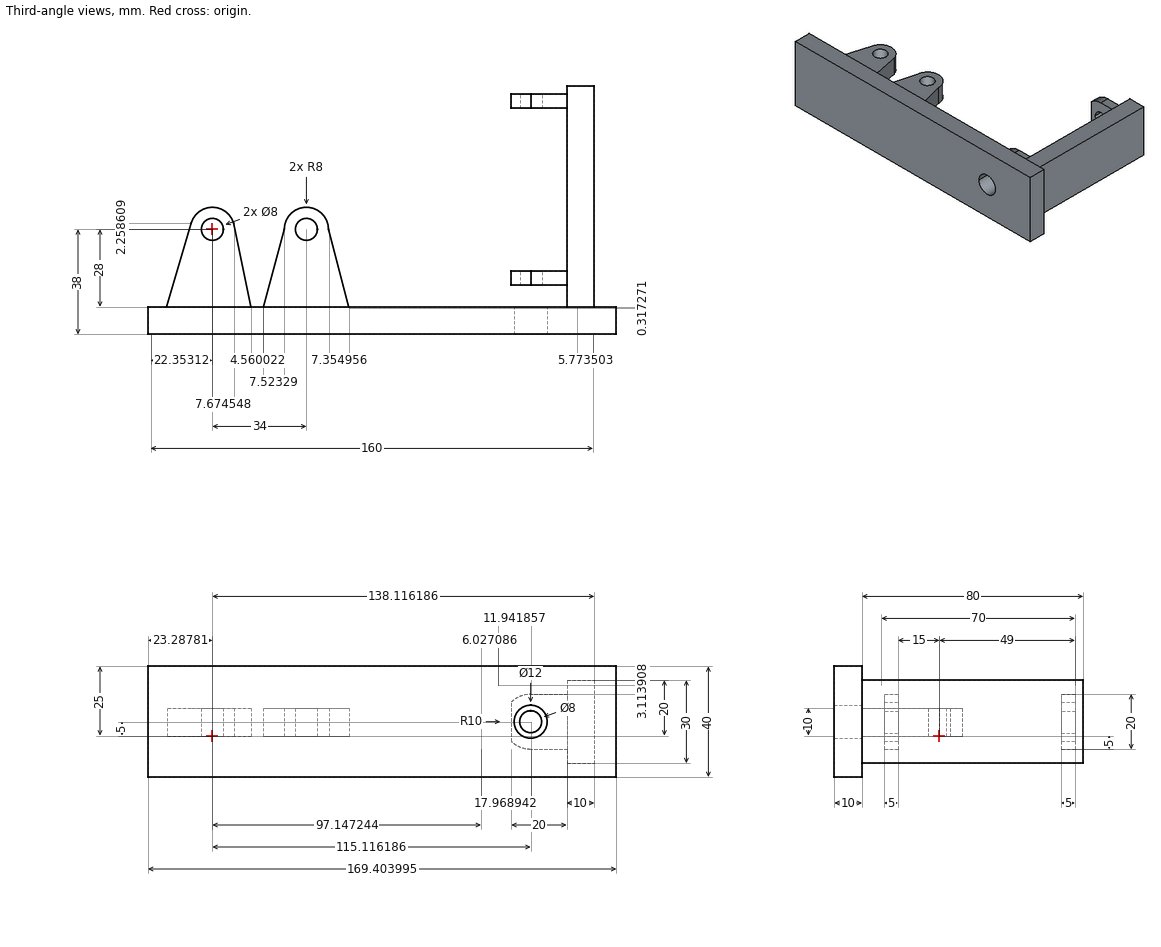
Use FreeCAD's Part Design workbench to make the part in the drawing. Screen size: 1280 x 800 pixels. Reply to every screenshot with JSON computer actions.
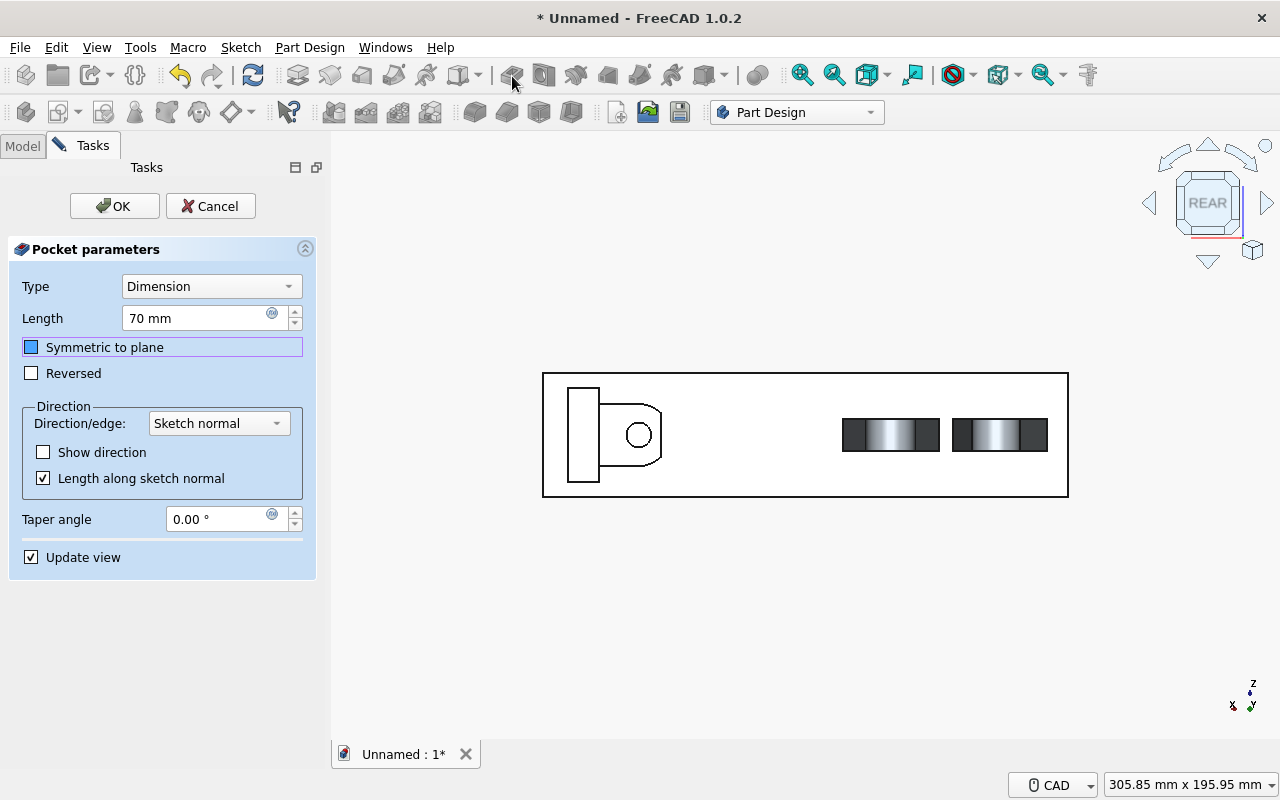
{"action": "left_click", "coordinate": [115, 206]}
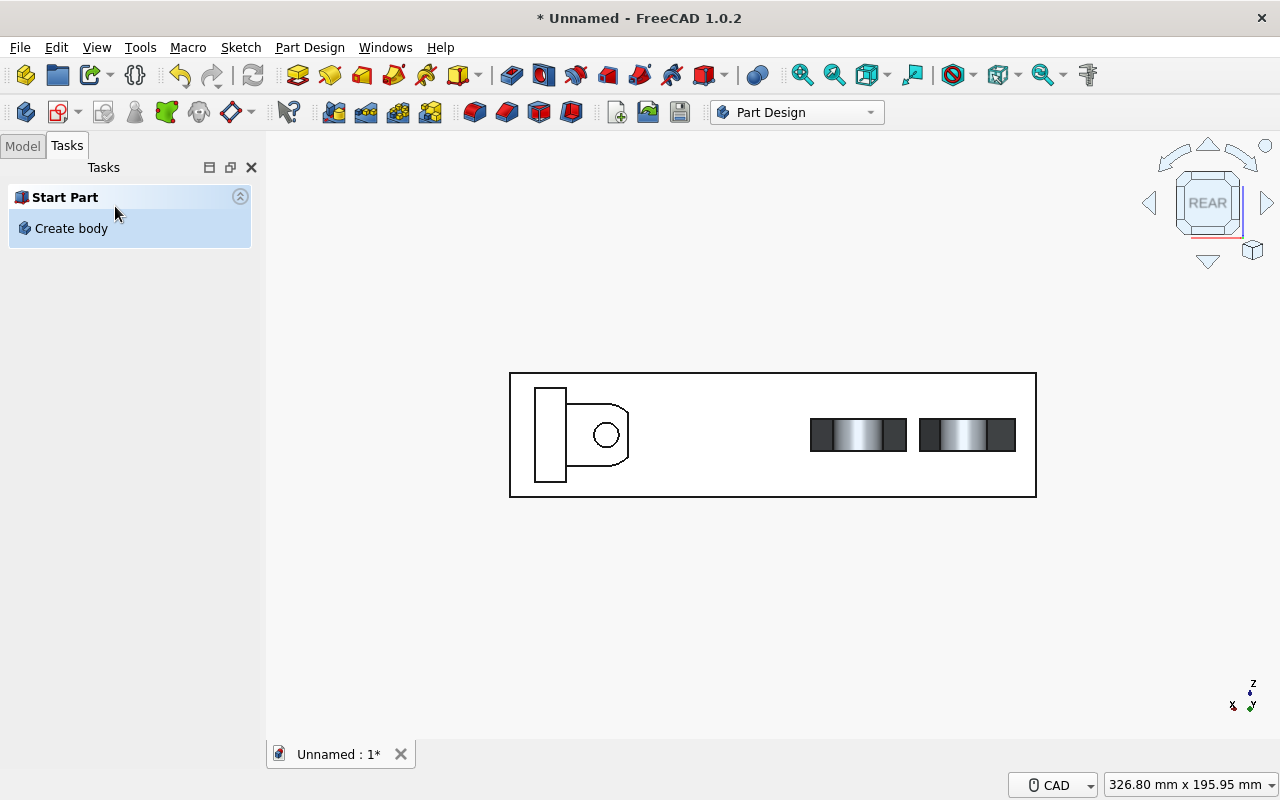
{"action": "left_click", "coordinate": [698, 434]}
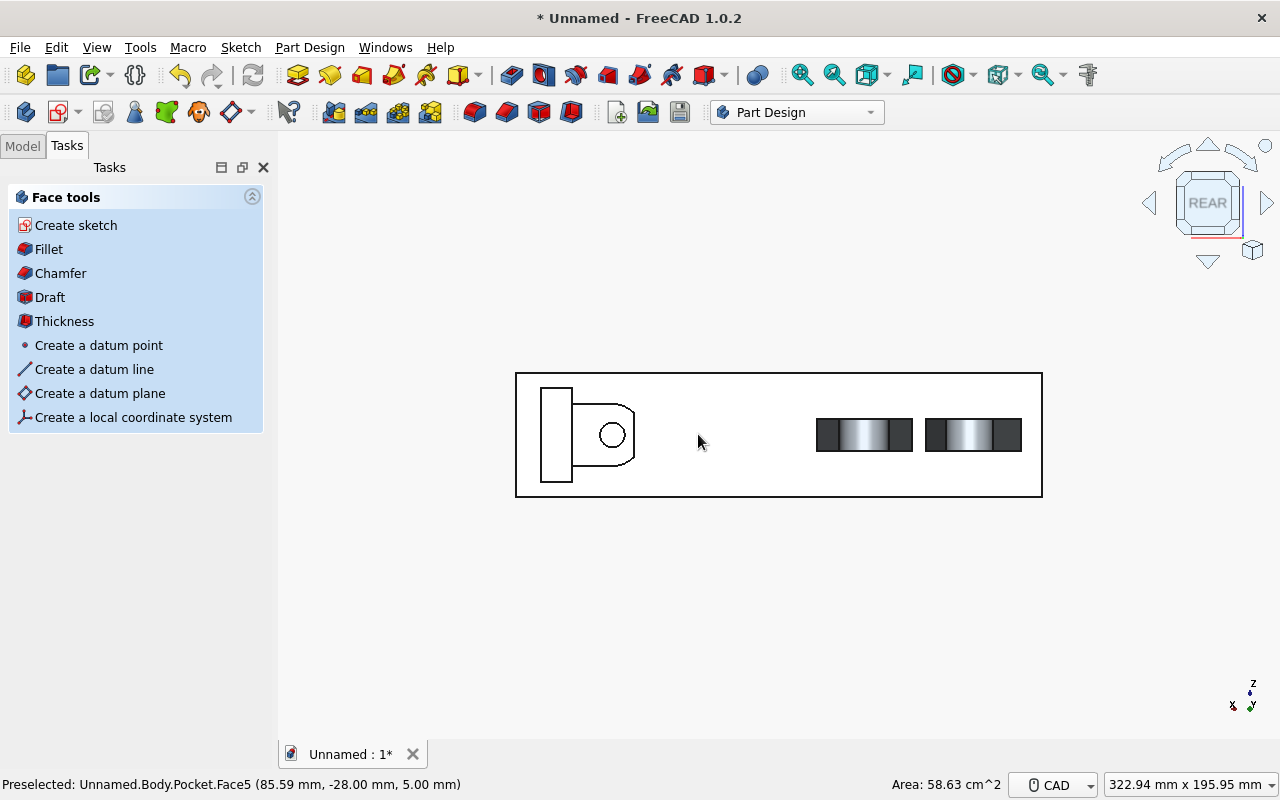
{"action": "left_click", "coordinate": [58, 112]}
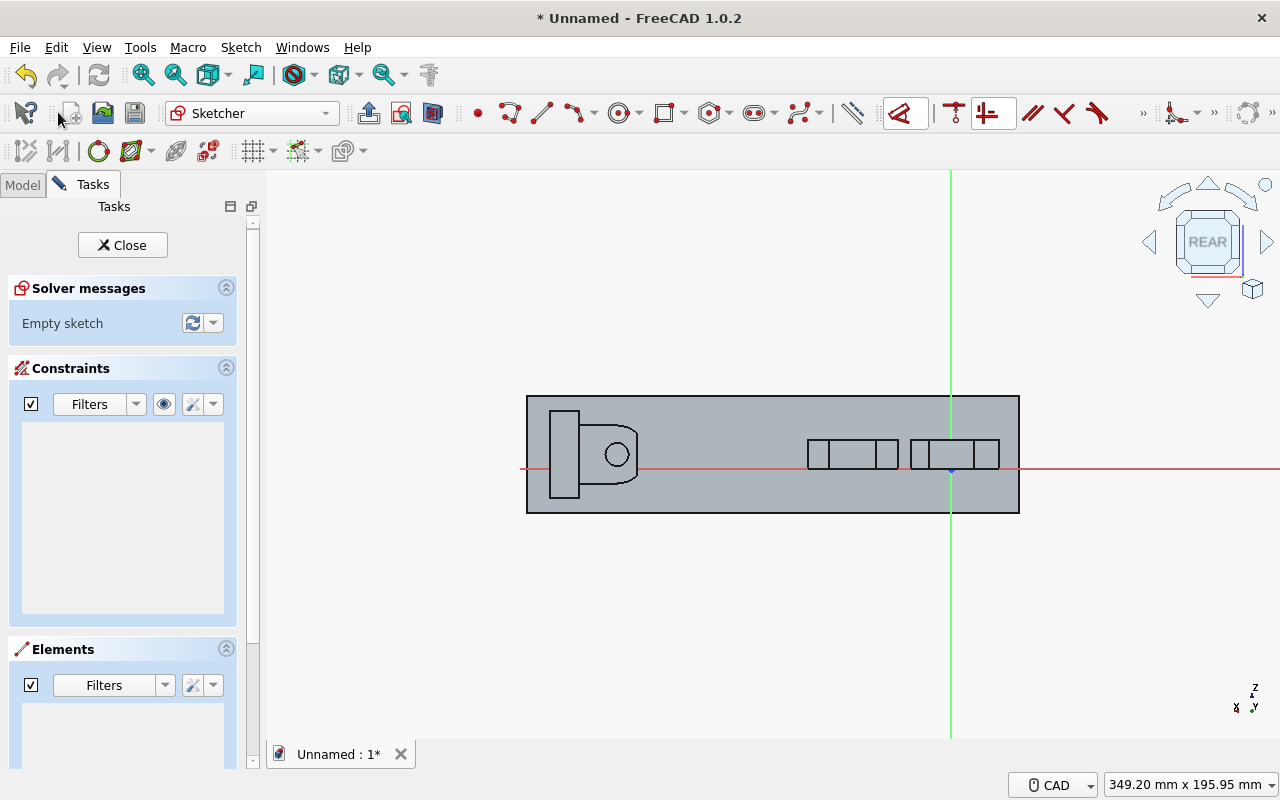
{"action": "scroll", "coordinate": [608, 455], "scroll_direction": "up", "scroll_amount": 12}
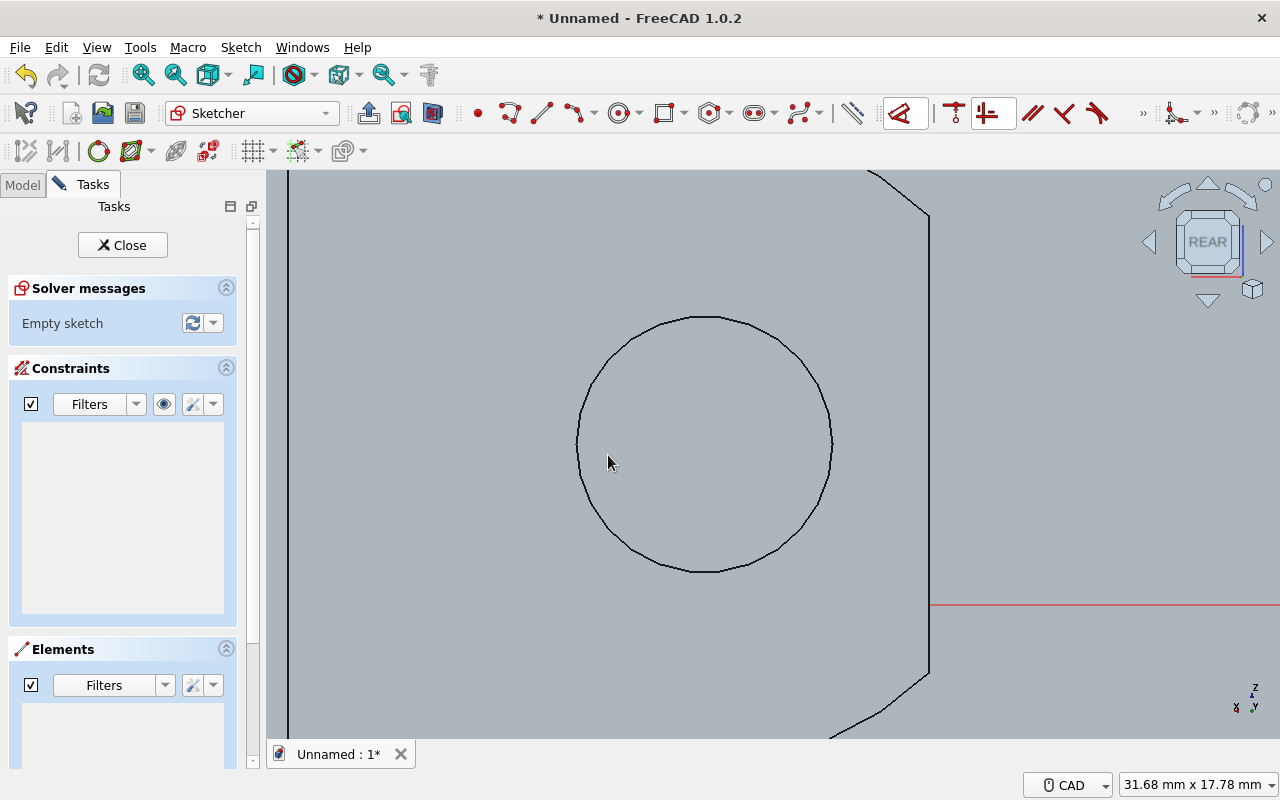
{"action": "left_click", "coordinate": [620, 114]}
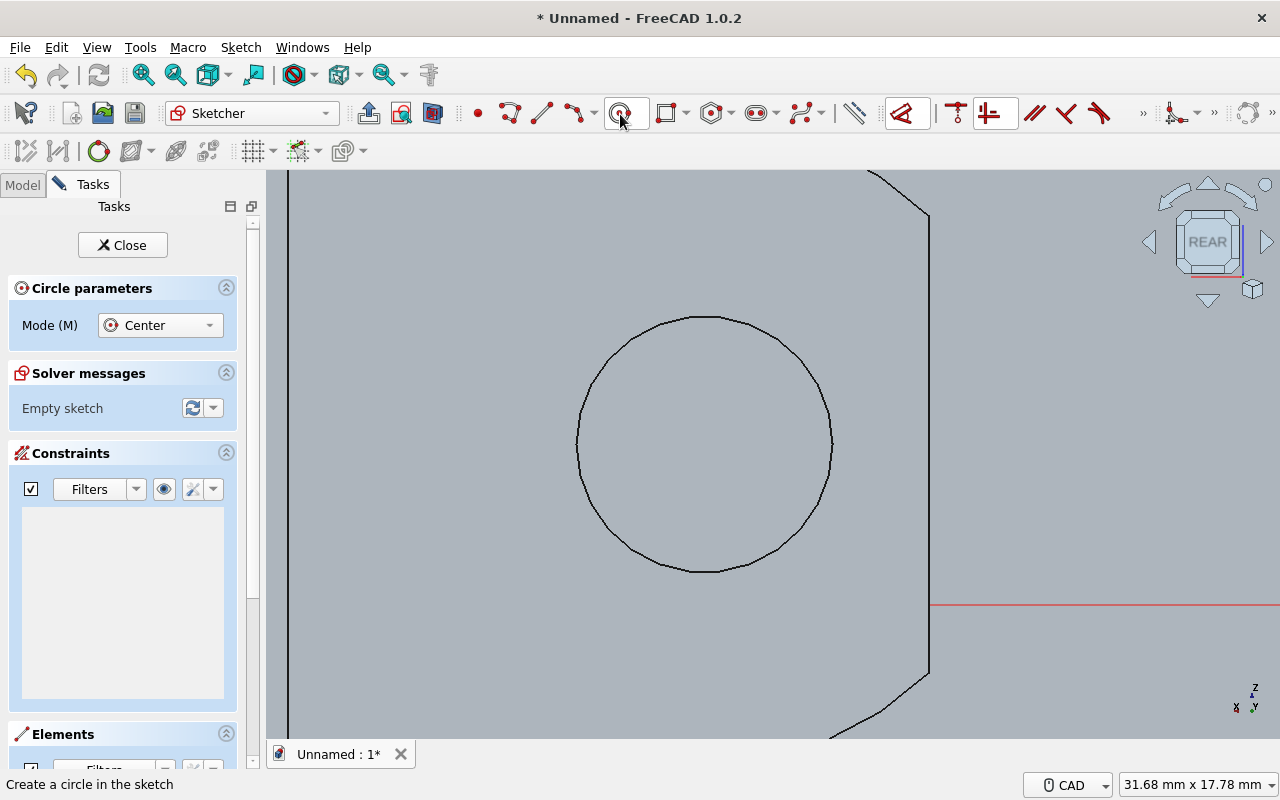
{"action": "left_click", "coordinate": [705, 444]}
{"action": "mouse_move", "coordinate": [840, 309]}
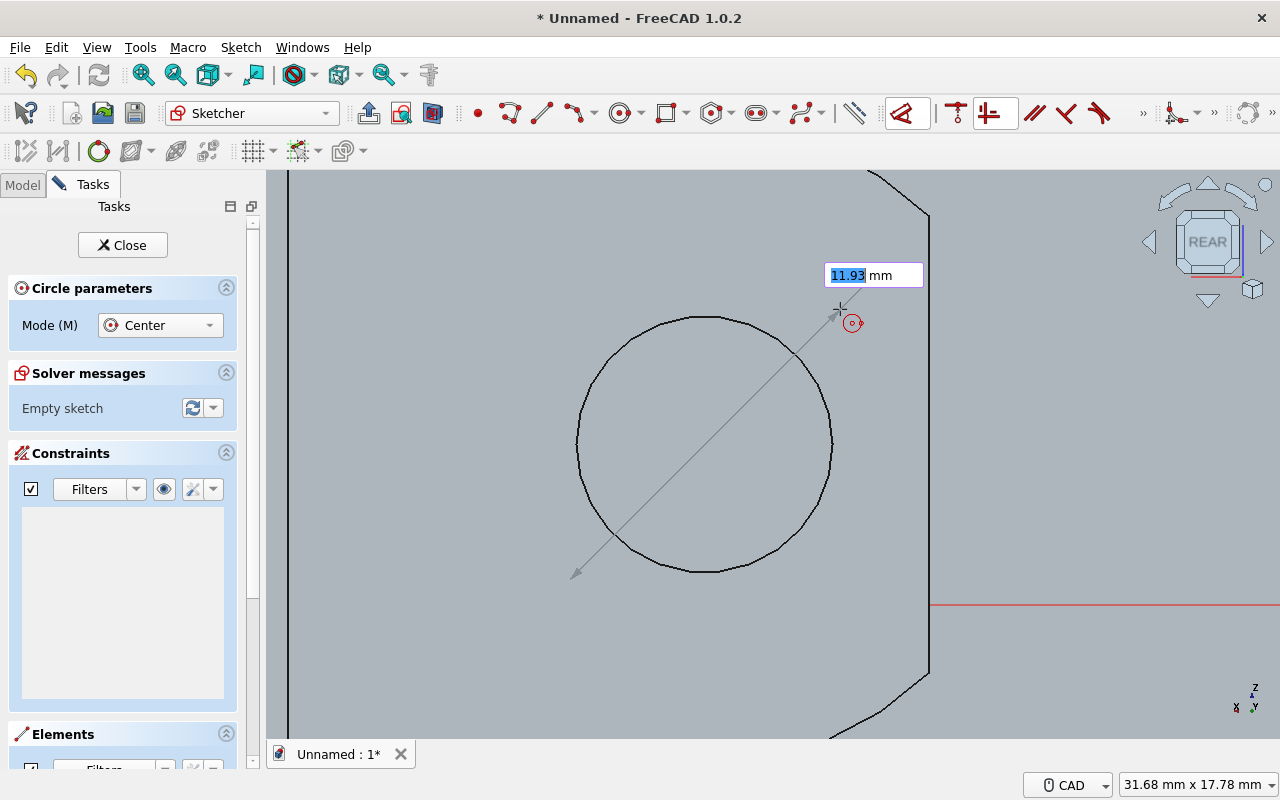
{"action": "type", "text": "12"}
{"action": "key", "text": "Return"}
{"action": "key", "text": "Escape"}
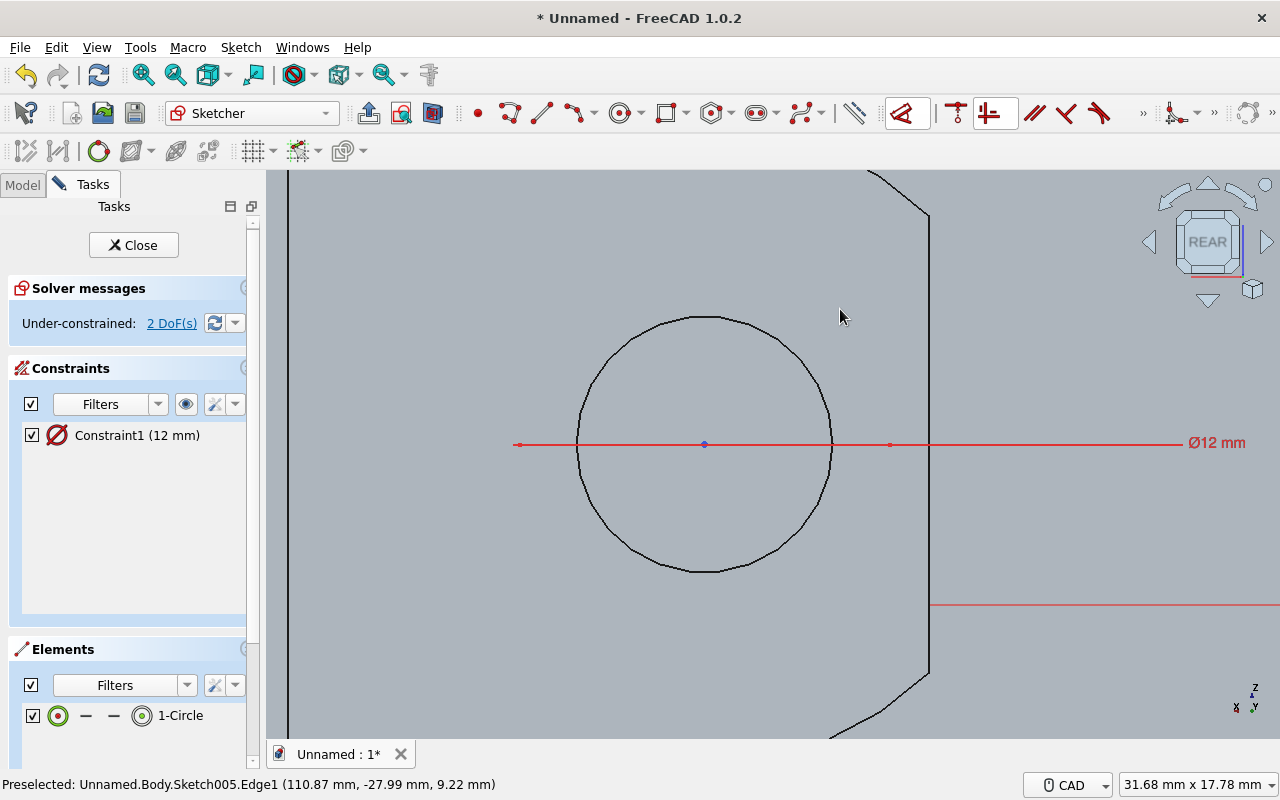
{"action": "left_click", "coordinate": [705, 445]}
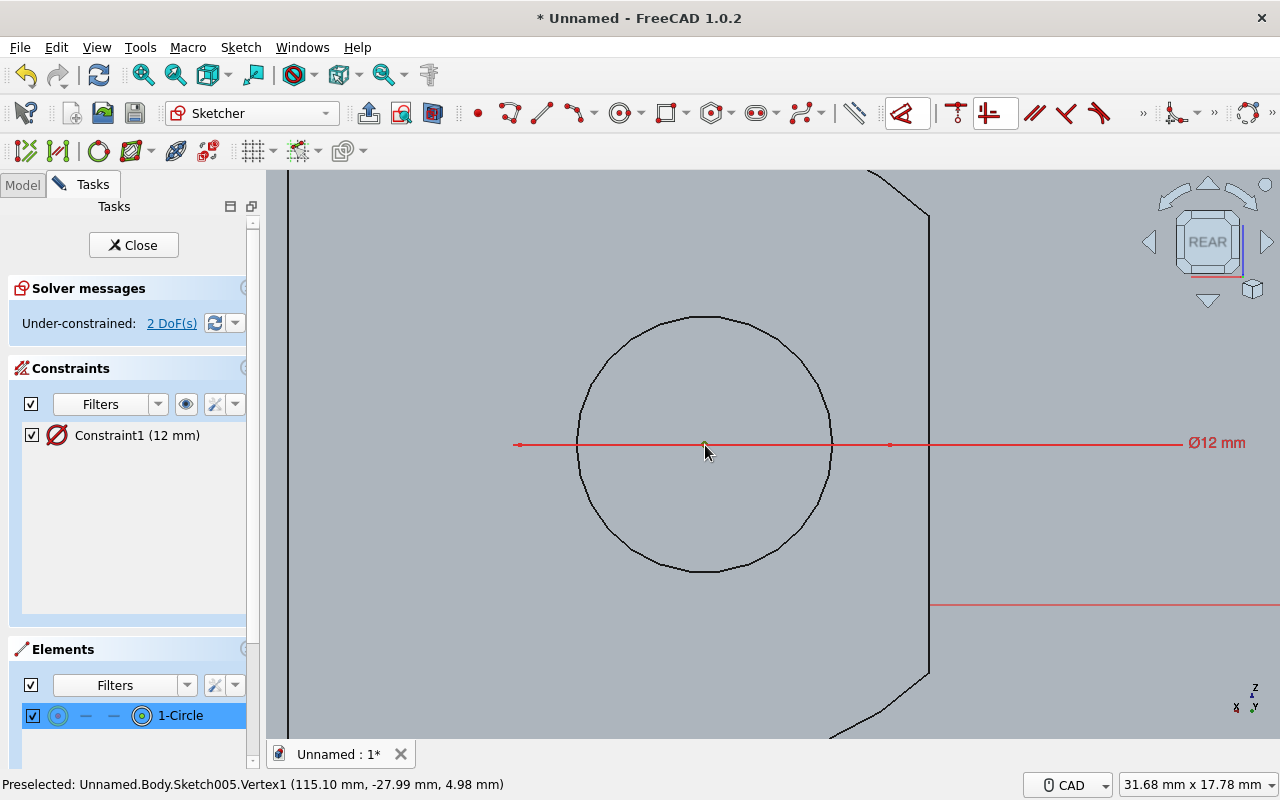
{"action": "key", "text": "i"}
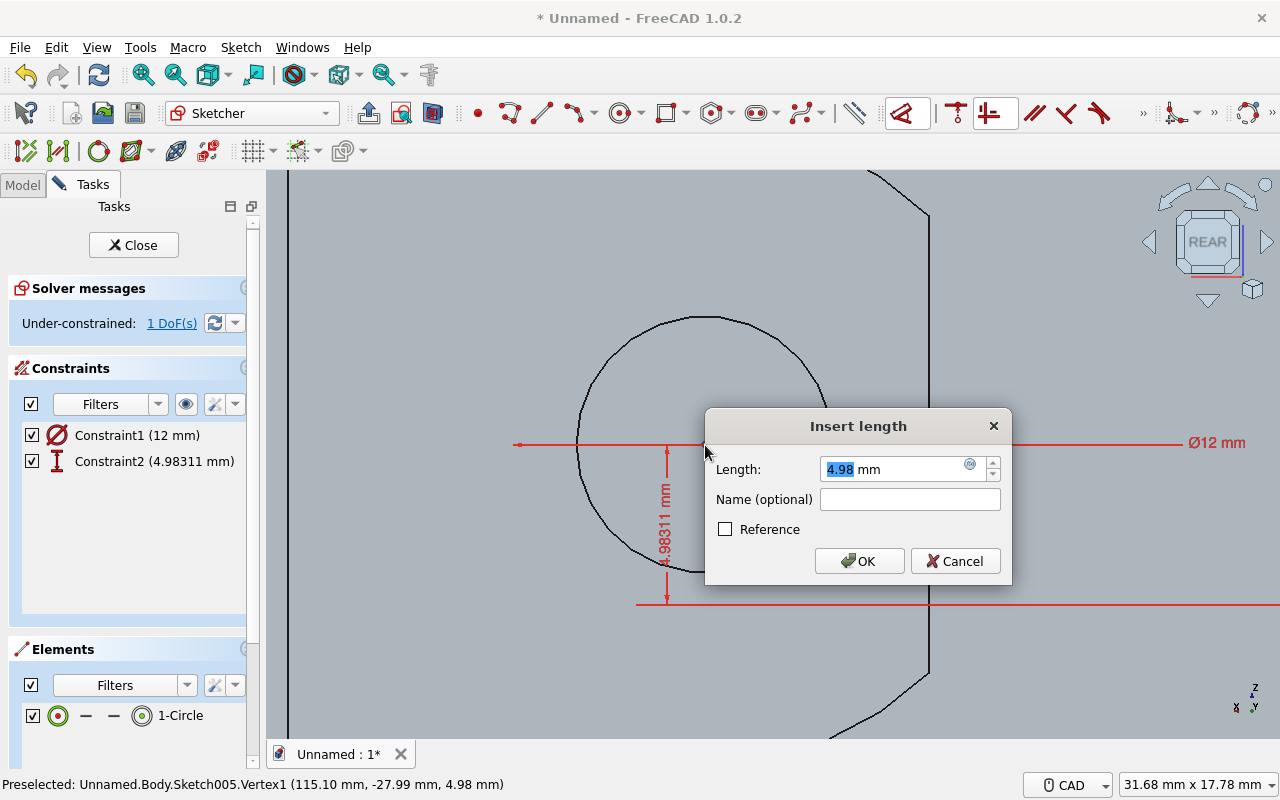
{"action": "type", "text": "5"}
{"action": "key", "text": "Return"}